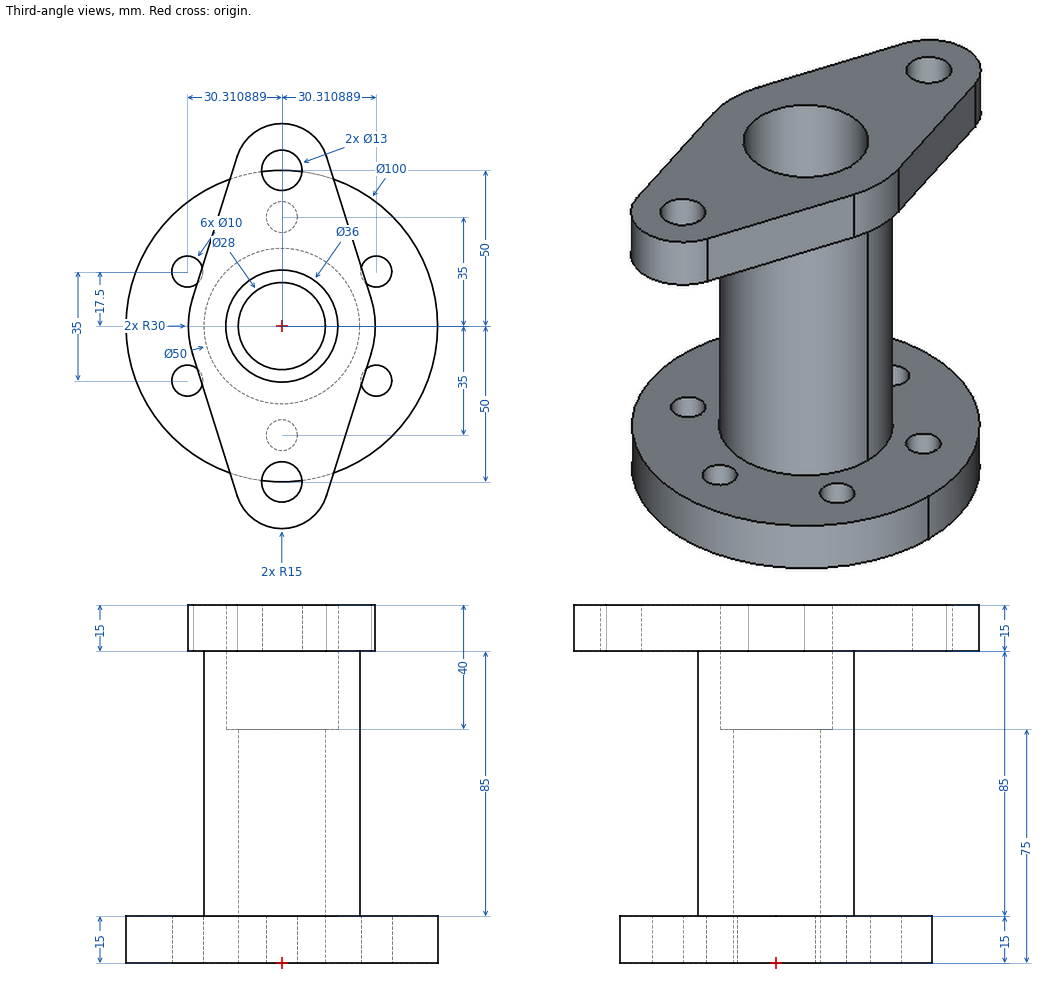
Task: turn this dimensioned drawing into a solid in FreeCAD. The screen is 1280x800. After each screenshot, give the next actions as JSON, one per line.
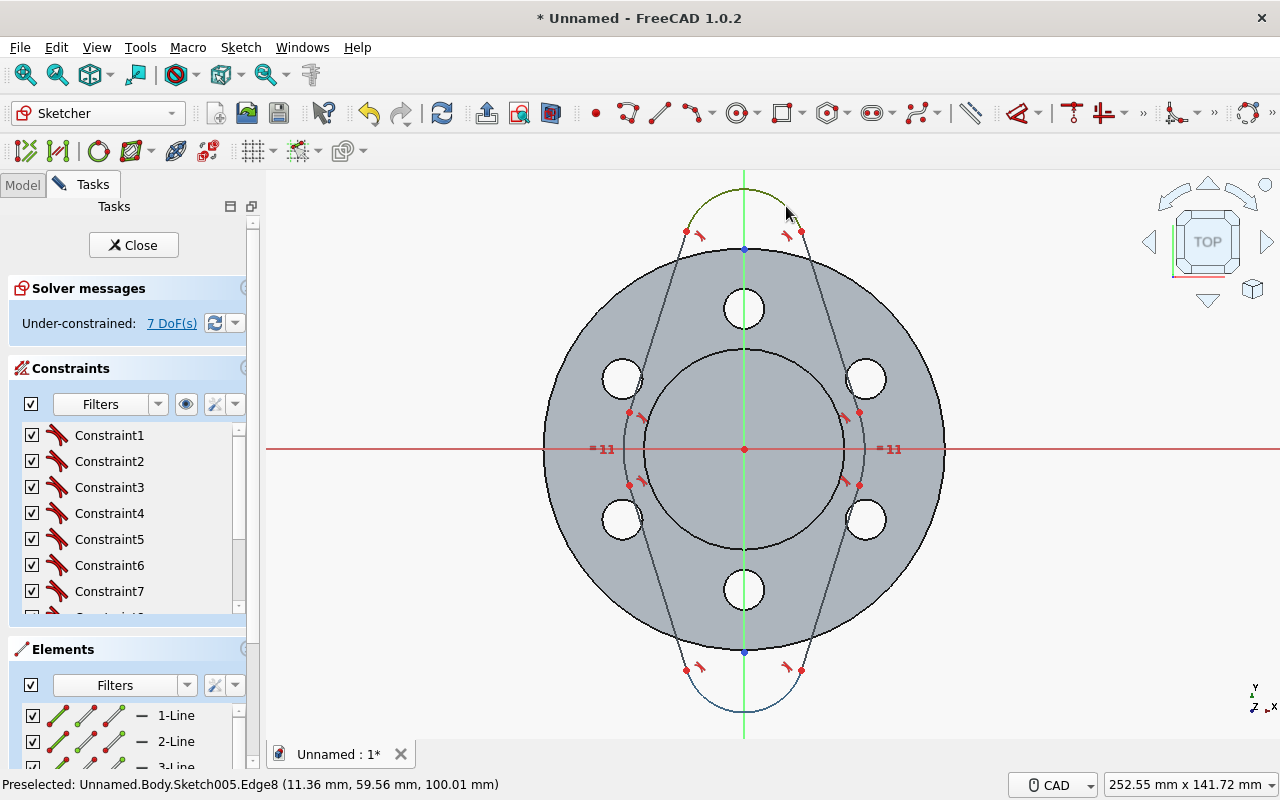
{"action": "key", "text": "e"}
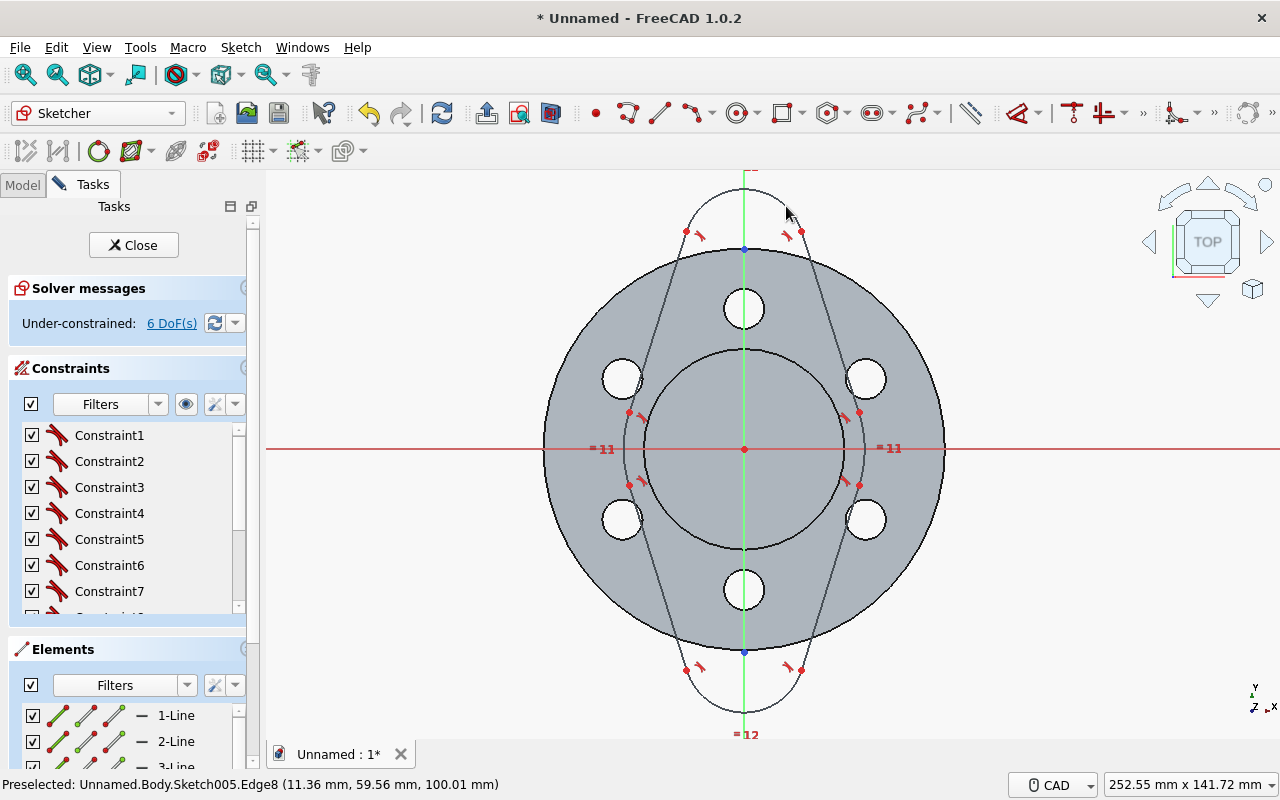
{"action": "left_click", "coordinate": [744, 652]}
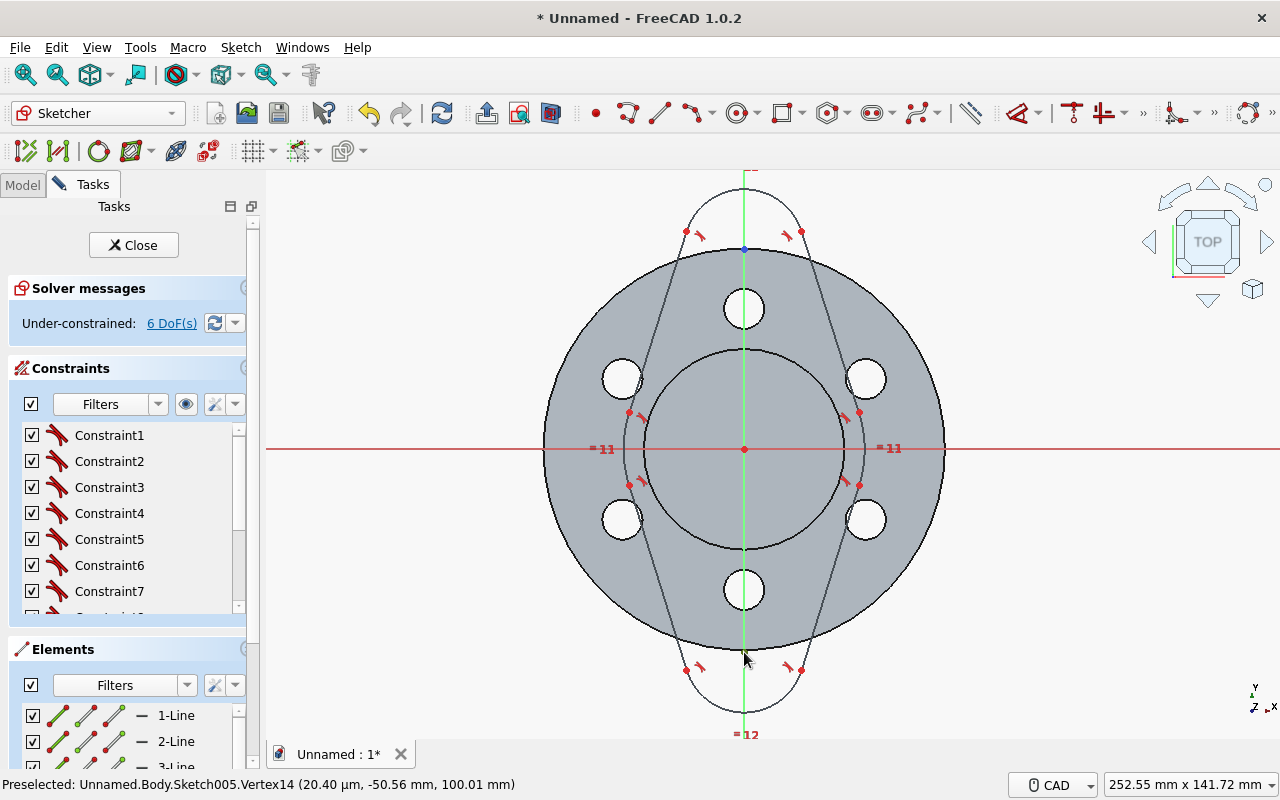
{"action": "left_click", "coordinate": [744, 674]}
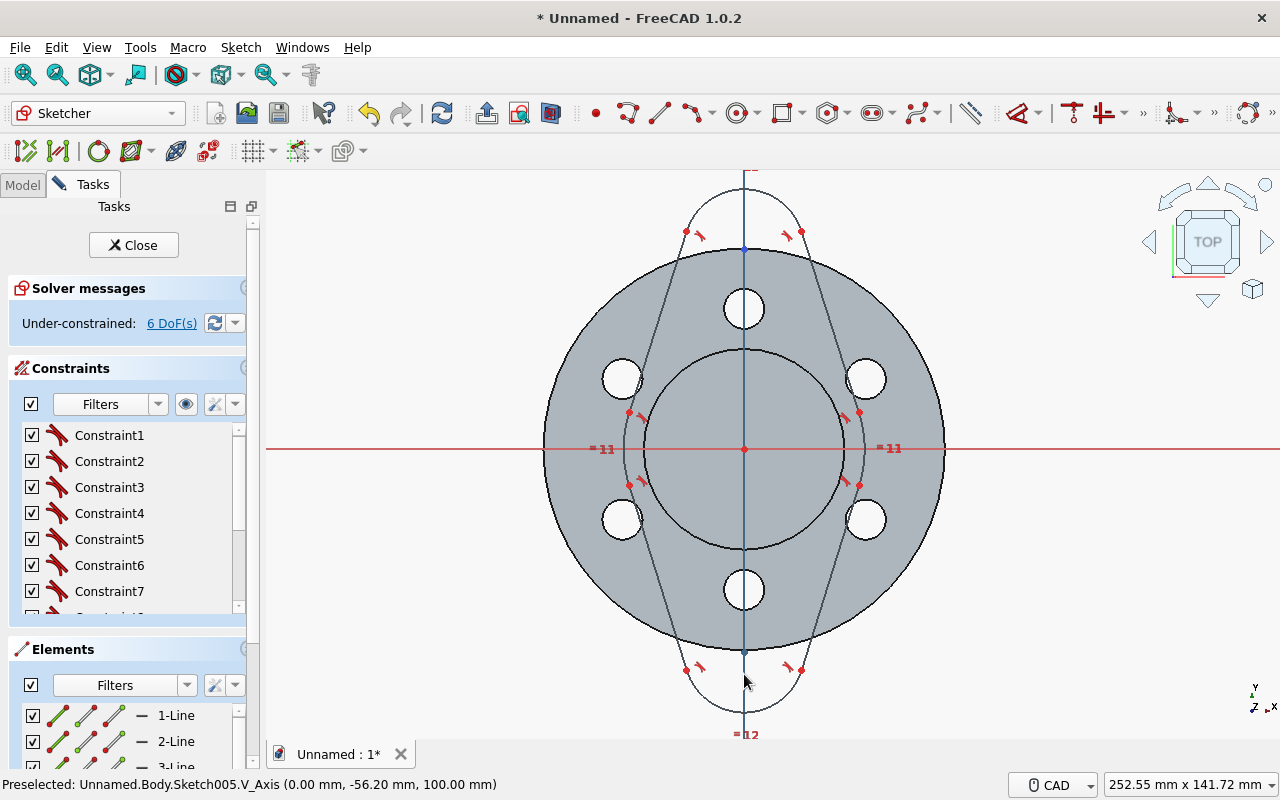
{"action": "left_click", "coordinate": [1072, 114]}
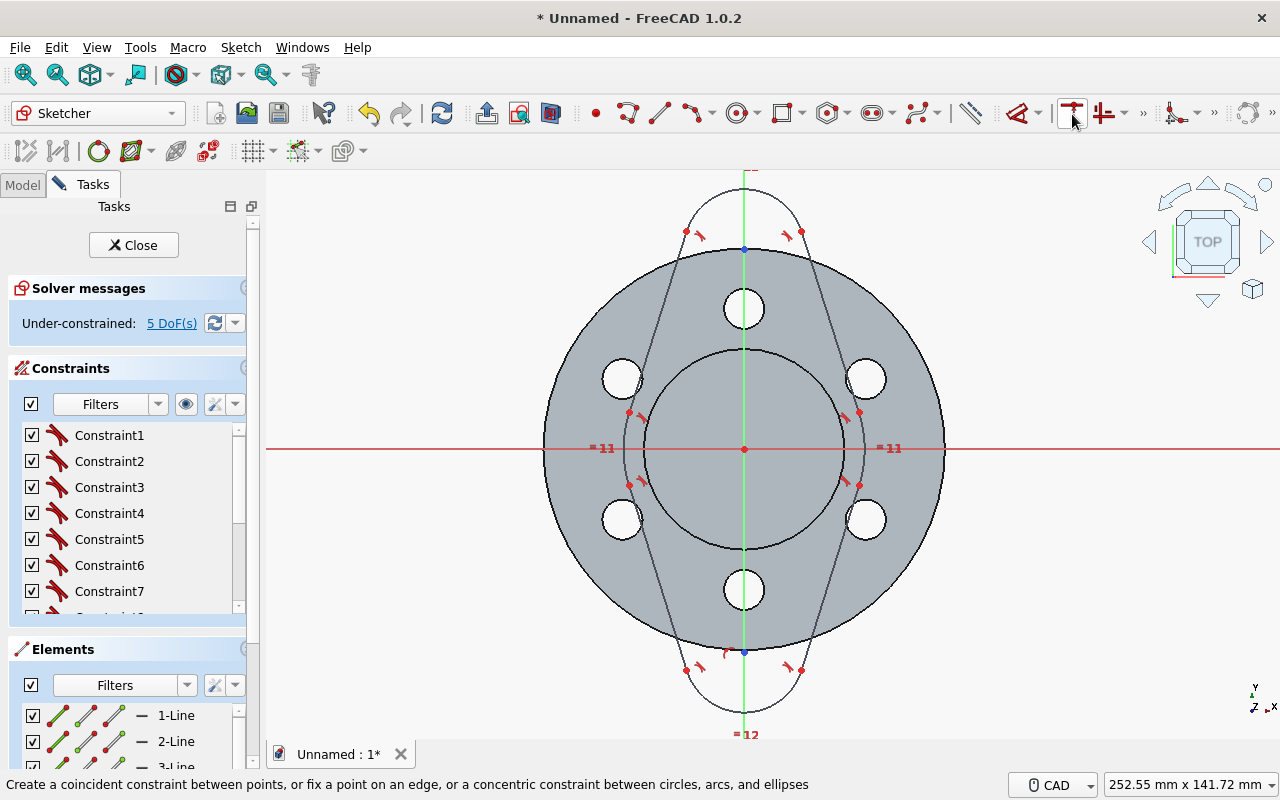
{"action": "left_click", "coordinate": [744, 249]}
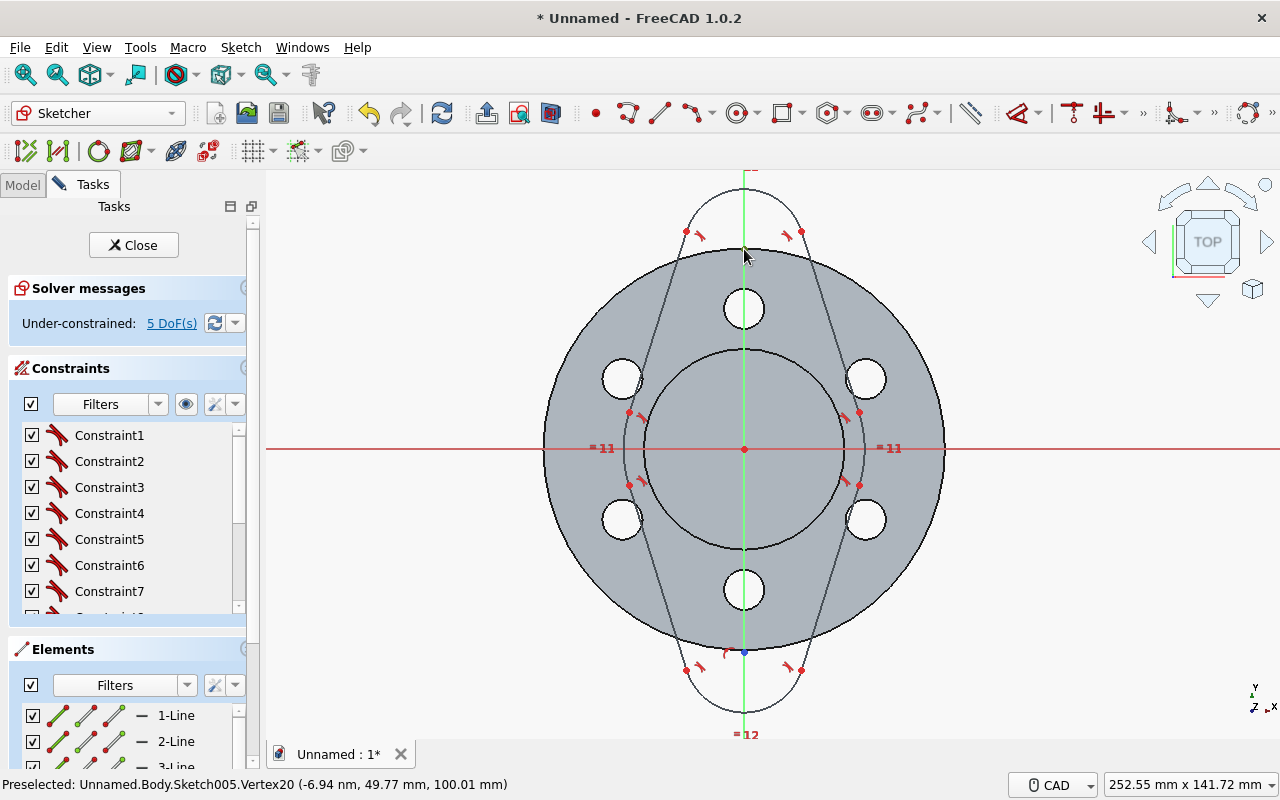
{"action": "left_click", "coordinate": [744, 674]}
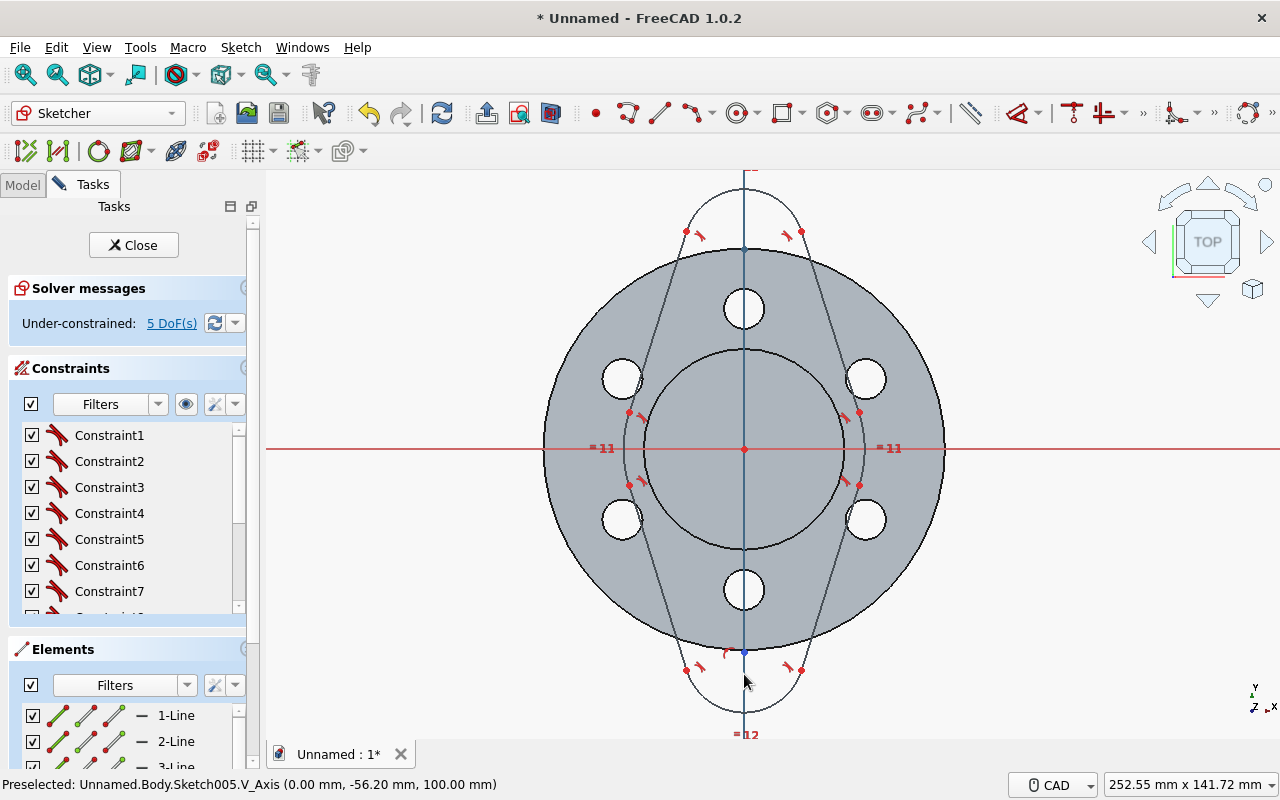
{"action": "left_click", "coordinate": [1072, 114]}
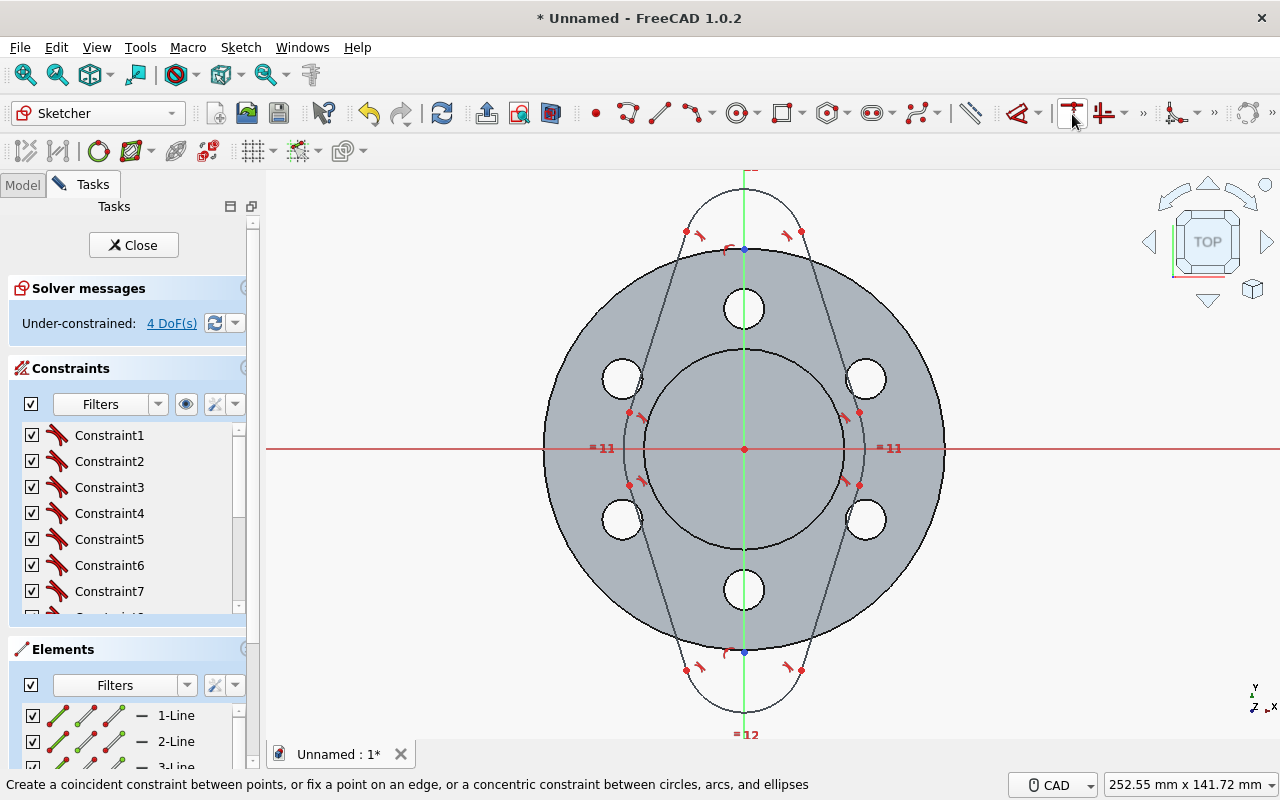
{"action": "left_click", "coordinate": [625, 434]}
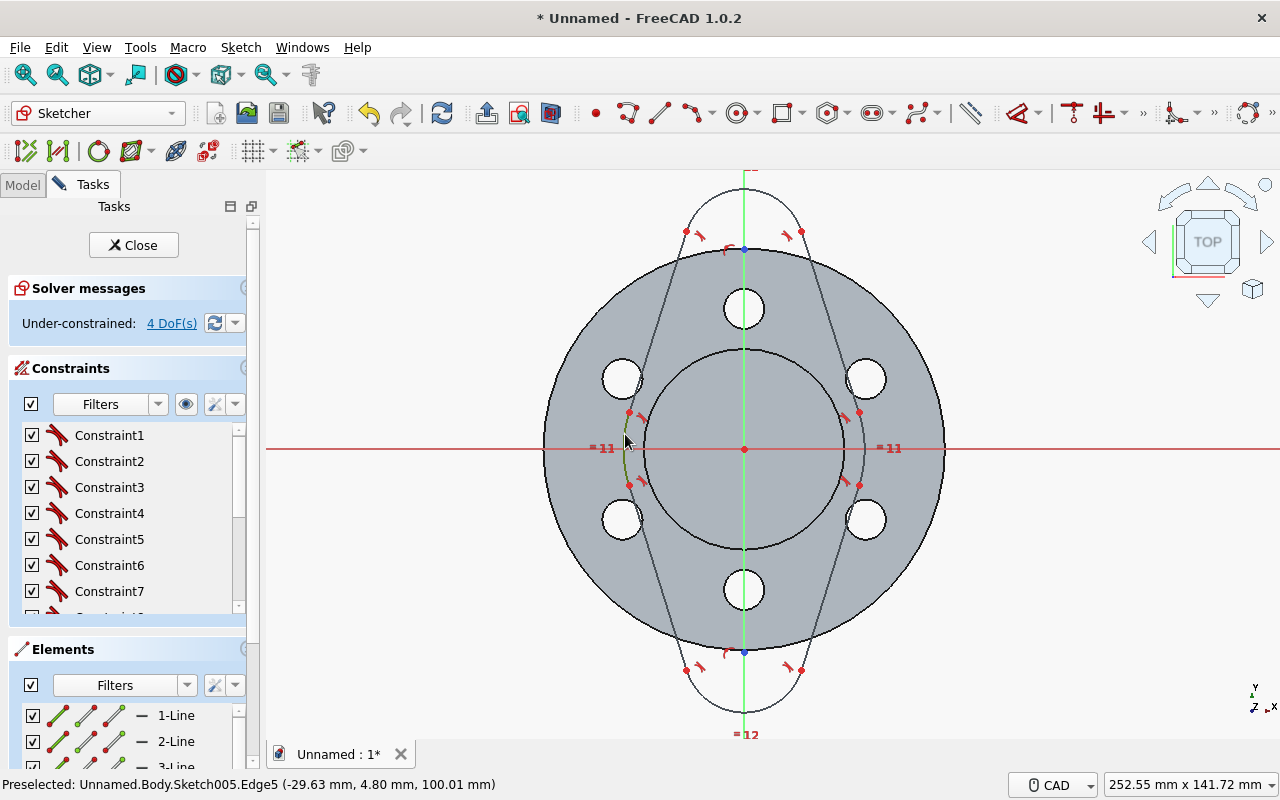
{"action": "key", "text": "k r"}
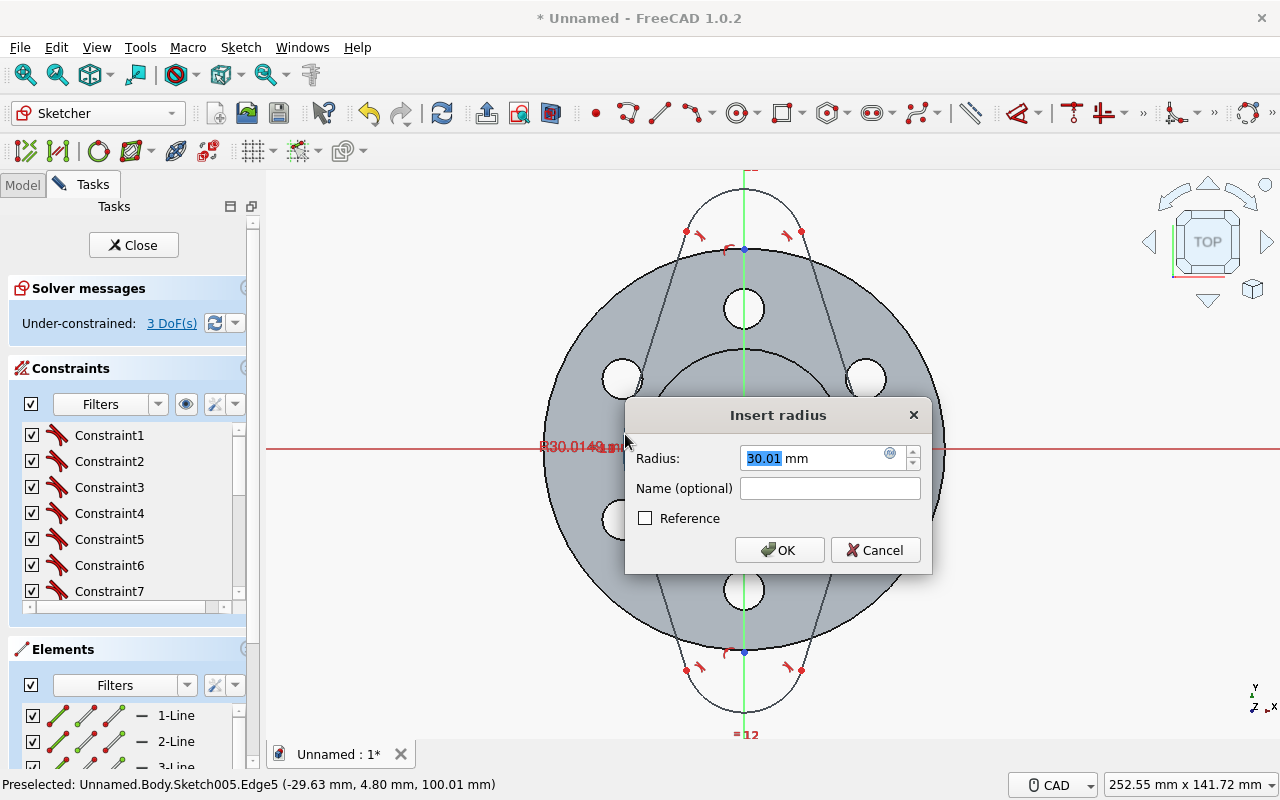
{"action": "type", "text": "30"}
{"action": "key", "text": "Return"}